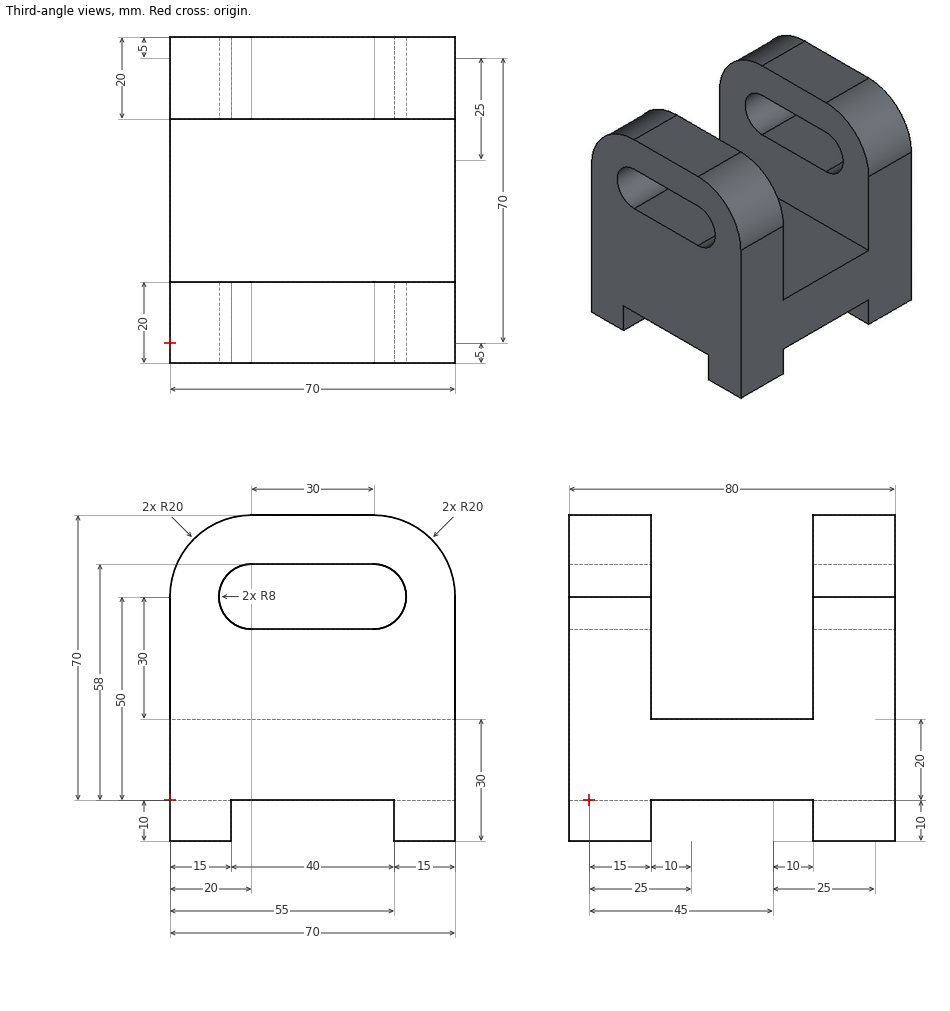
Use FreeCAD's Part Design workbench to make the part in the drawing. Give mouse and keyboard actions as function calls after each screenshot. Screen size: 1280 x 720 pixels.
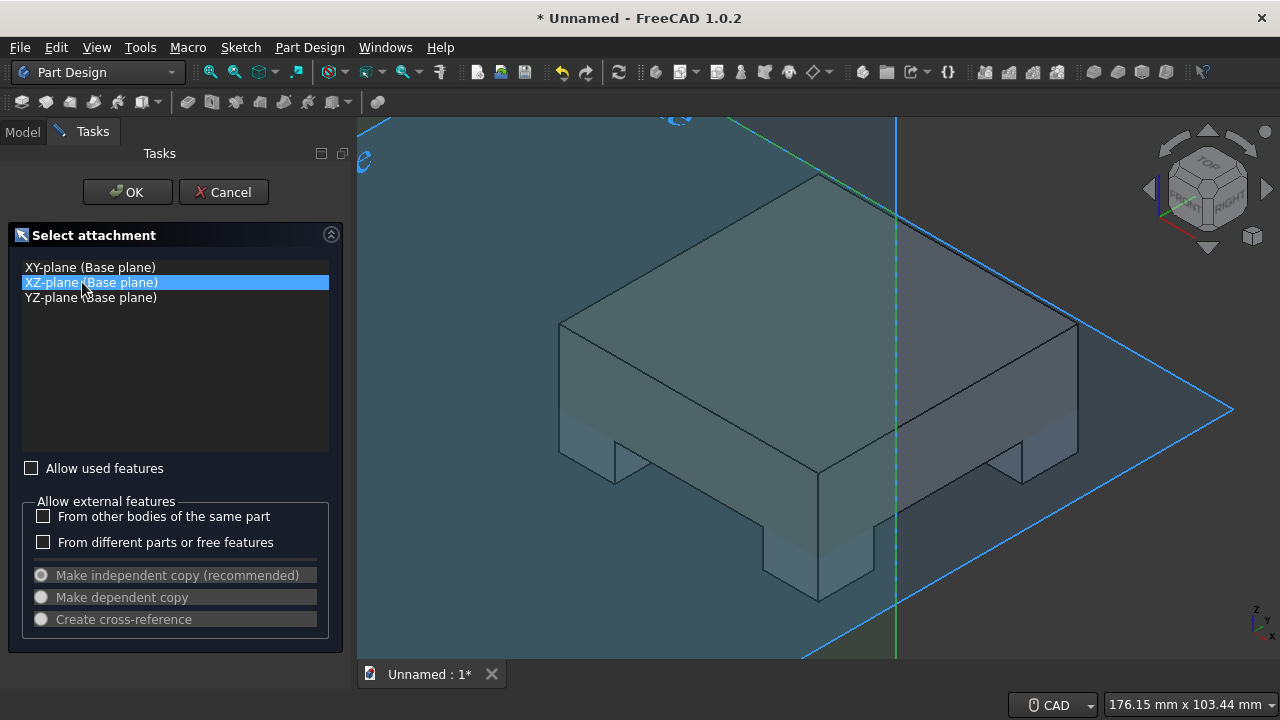
click(128, 192)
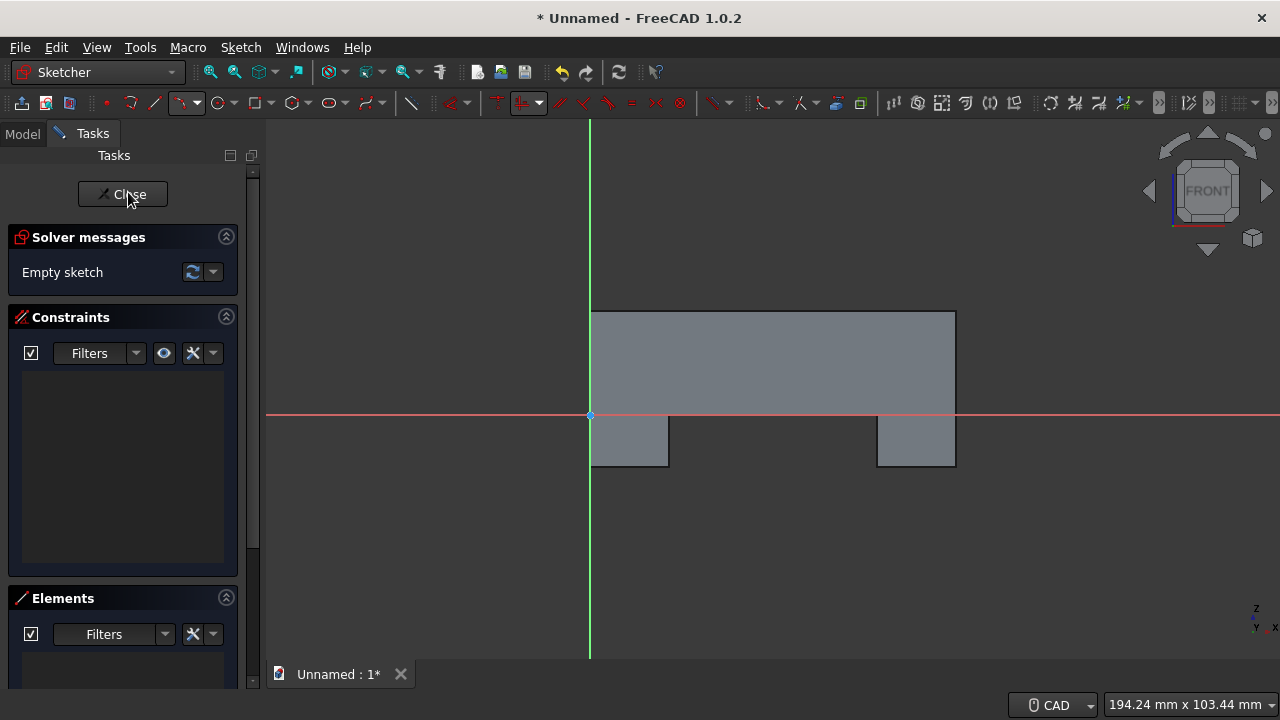
scroll(912, 389, up, 2)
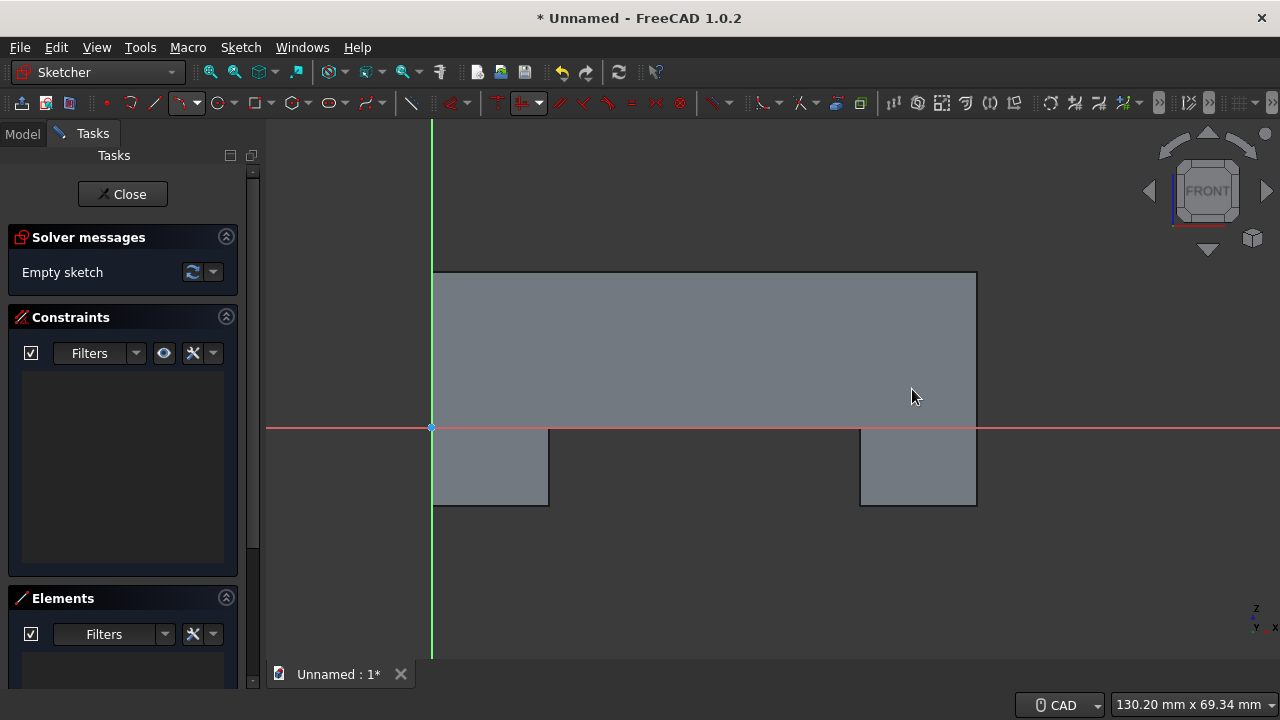
key(g)
key(m)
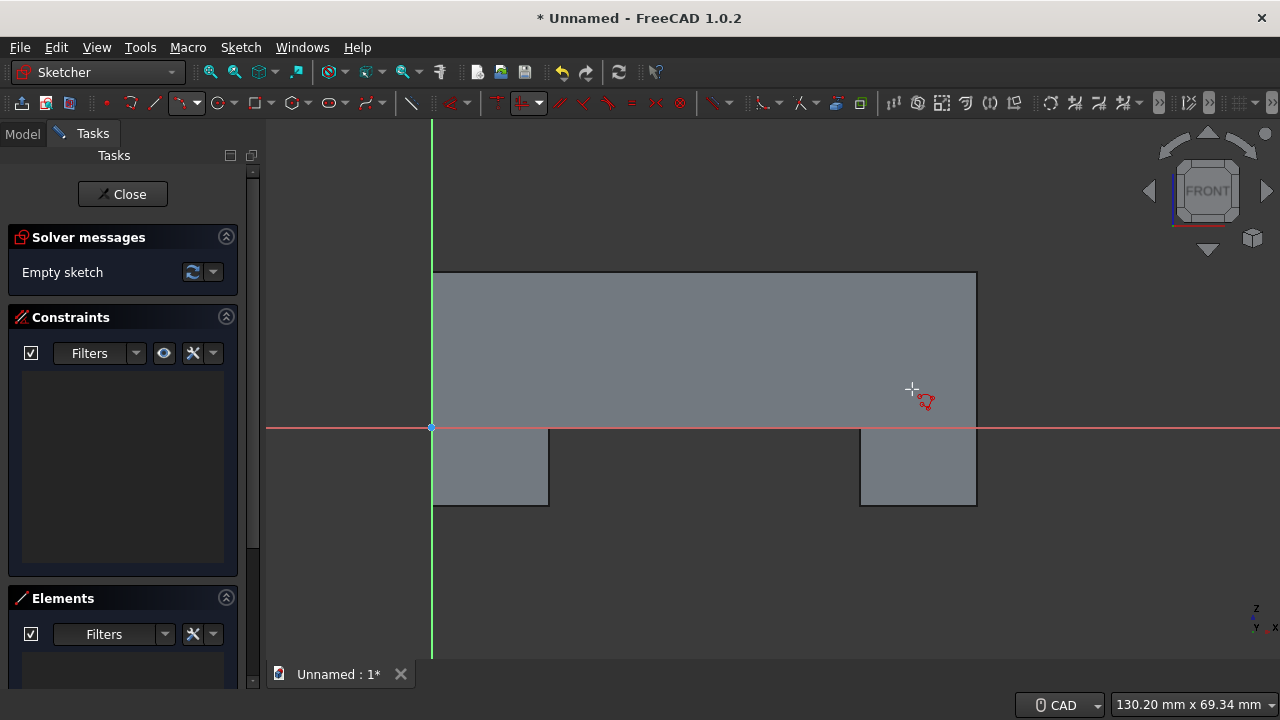
click(432, 506)
click(549, 506)
click(549, 428)
click(860, 419)
click(860, 506)
click(977, 506)
click(977, 272)
click(441, 272)
click(432, 507)
key(Escape)
key(Escape)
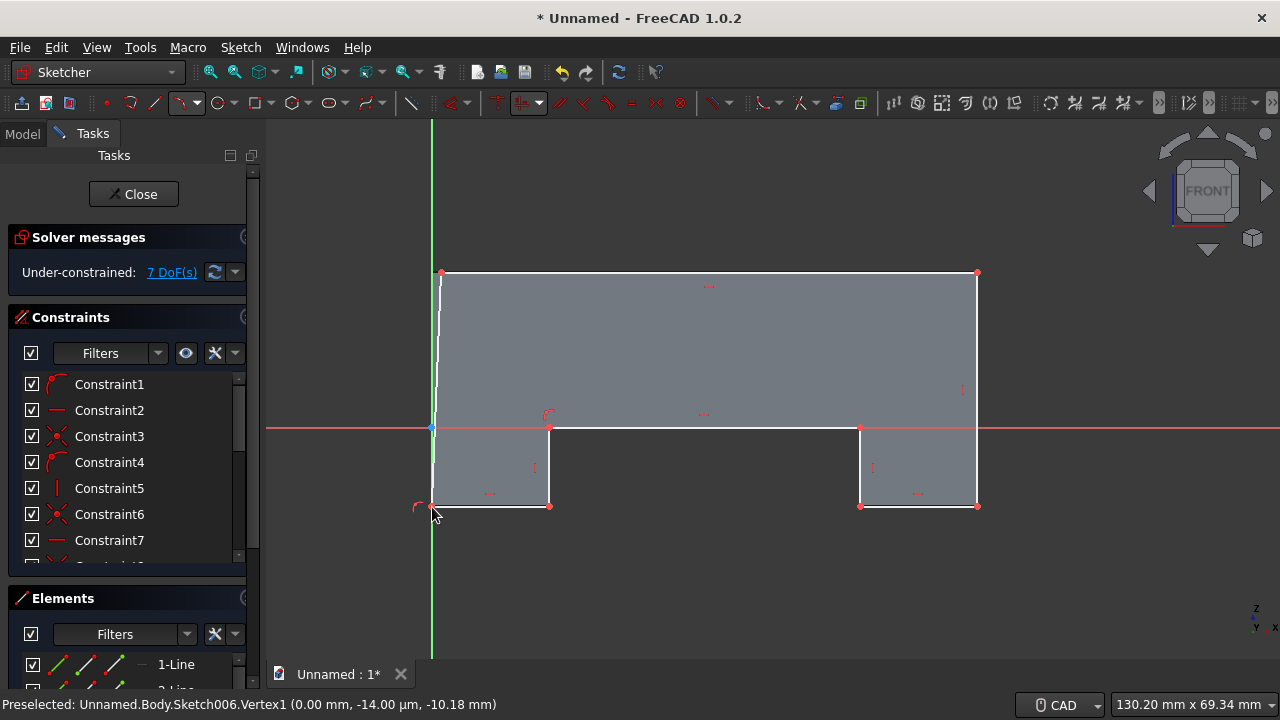
scroll(435, 437, up, 3)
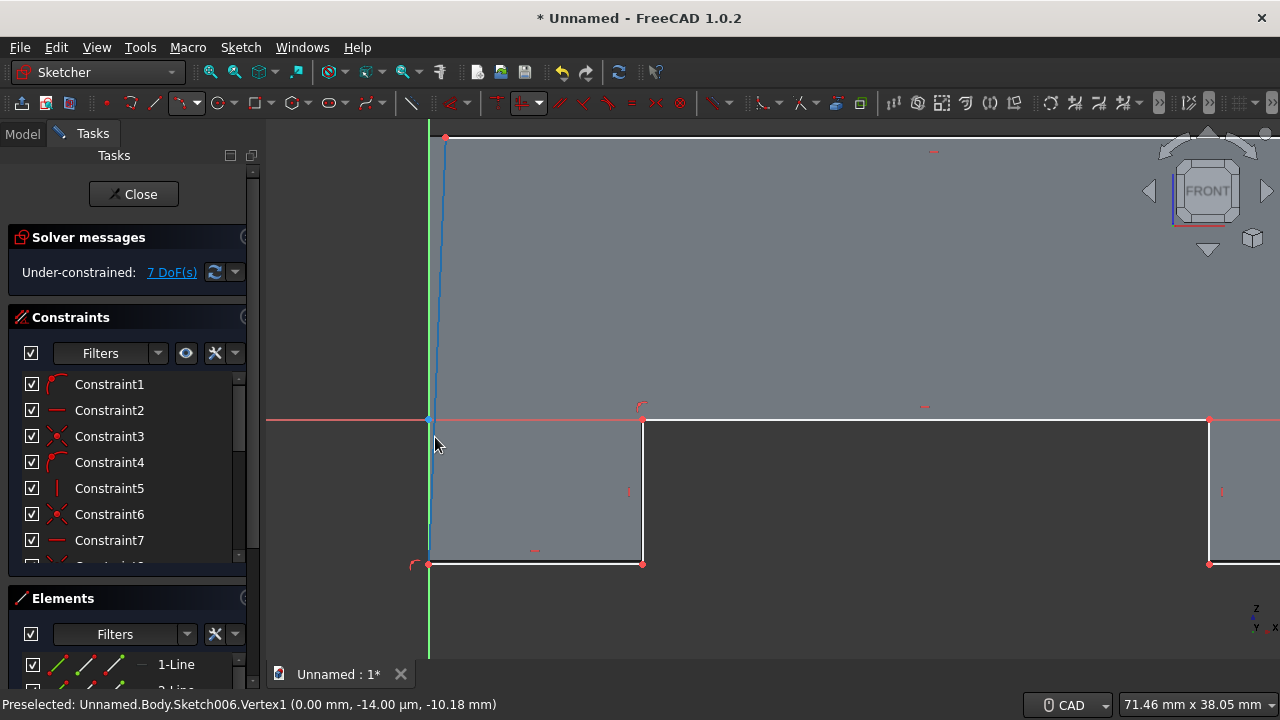
click(434, 436)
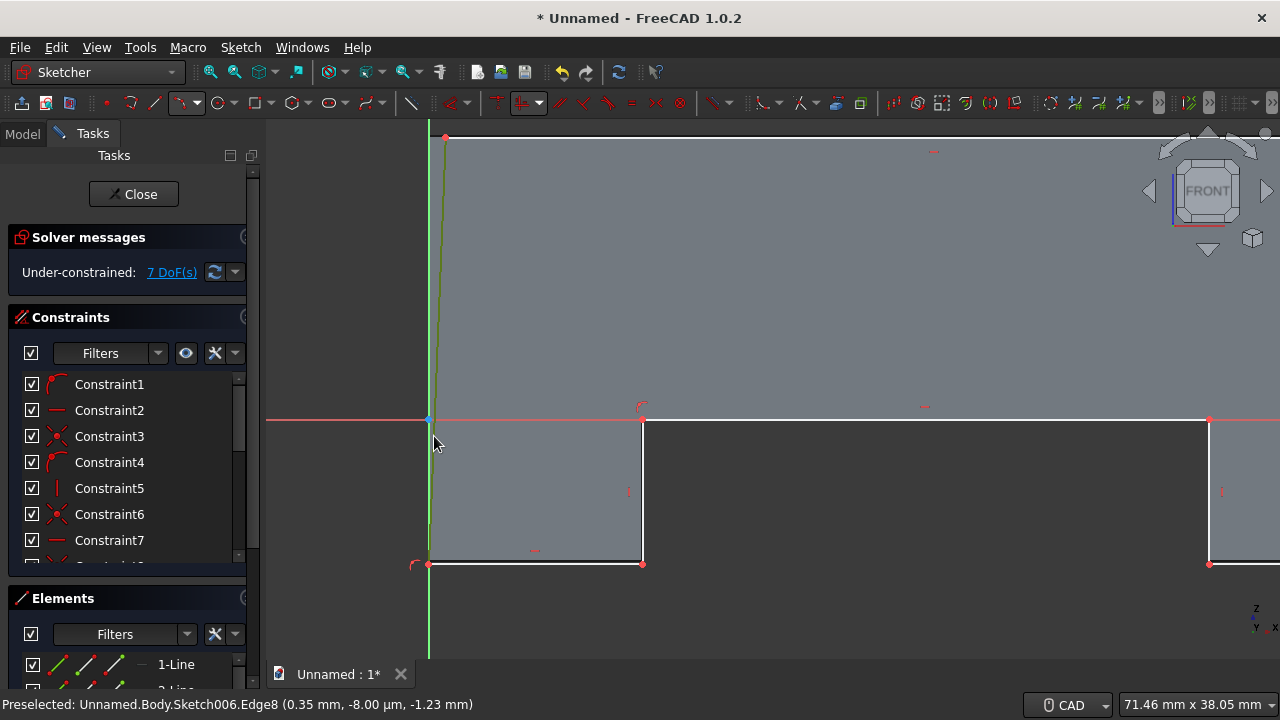
key(v)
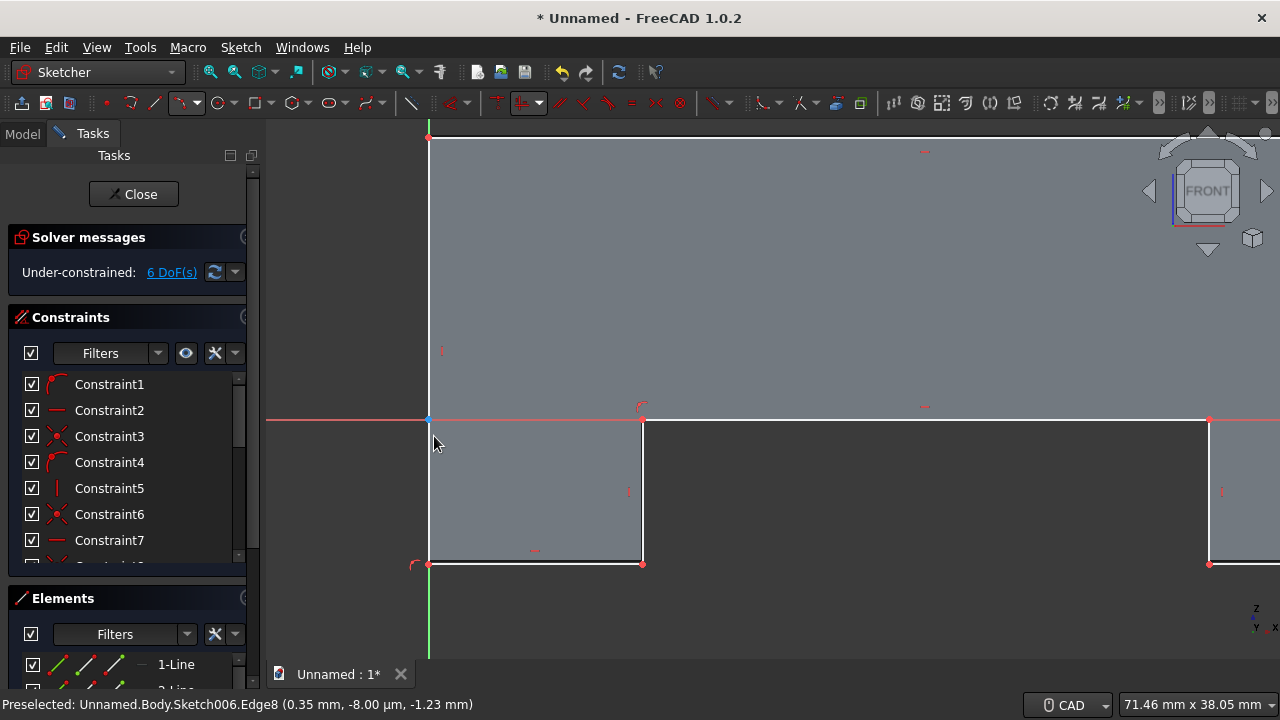
click(450, 104)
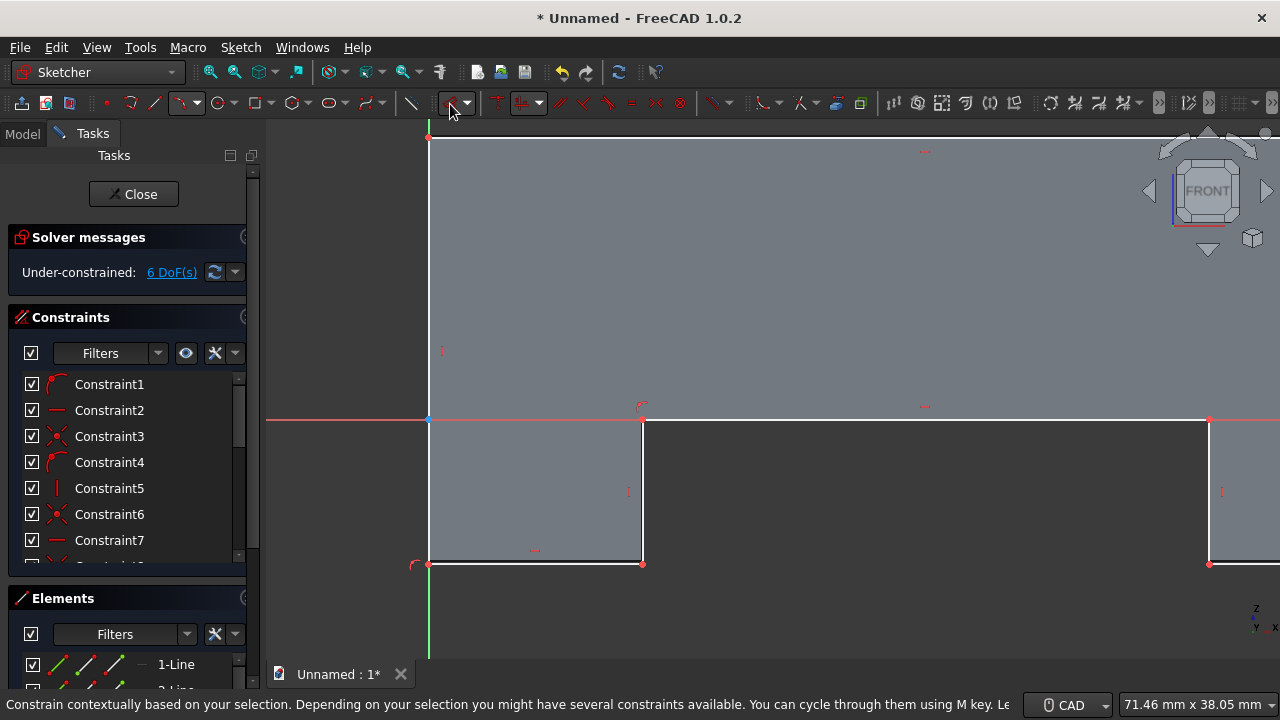
click(493, 564)
click(536, 598)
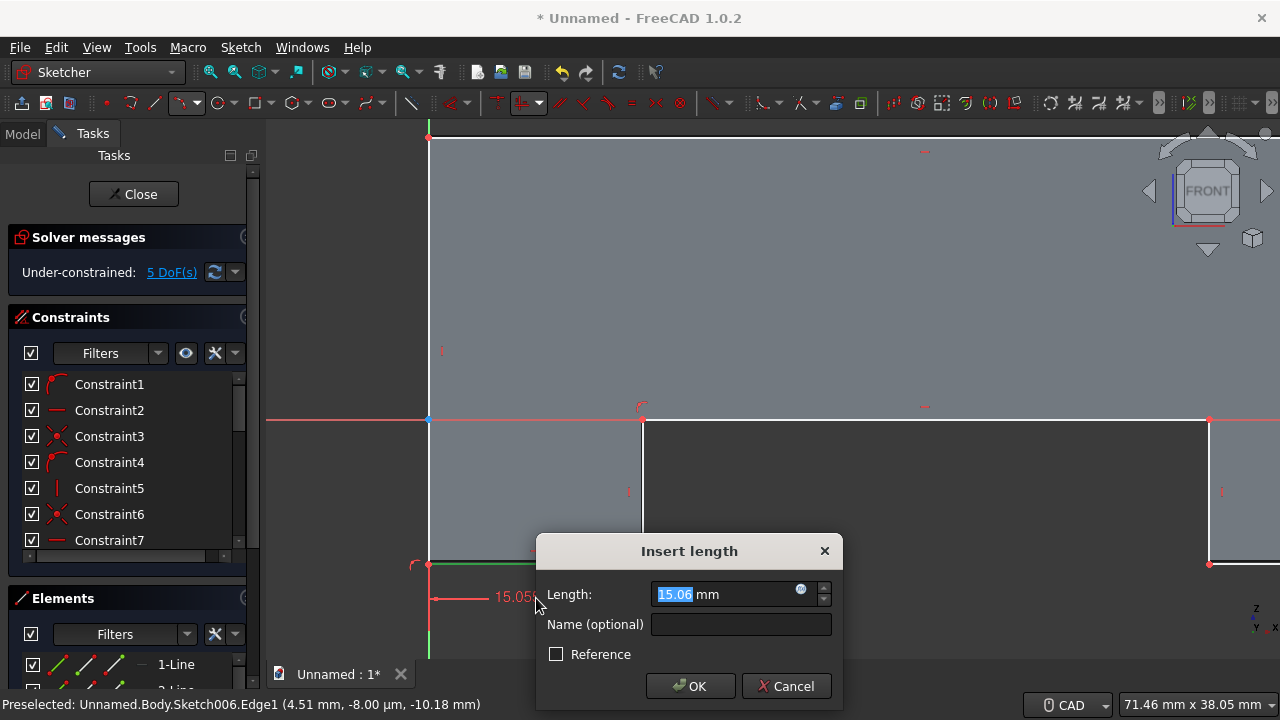
text(15)
key(Return)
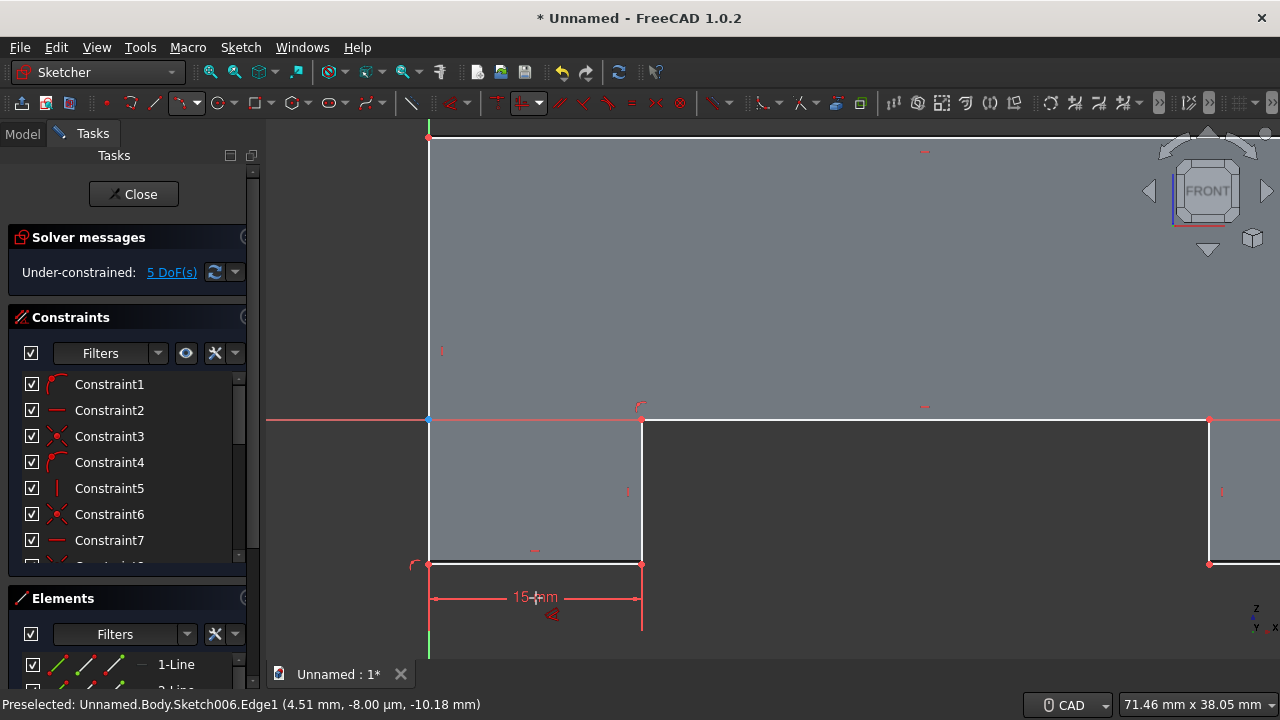
click(642, 521)
click(608, 492)